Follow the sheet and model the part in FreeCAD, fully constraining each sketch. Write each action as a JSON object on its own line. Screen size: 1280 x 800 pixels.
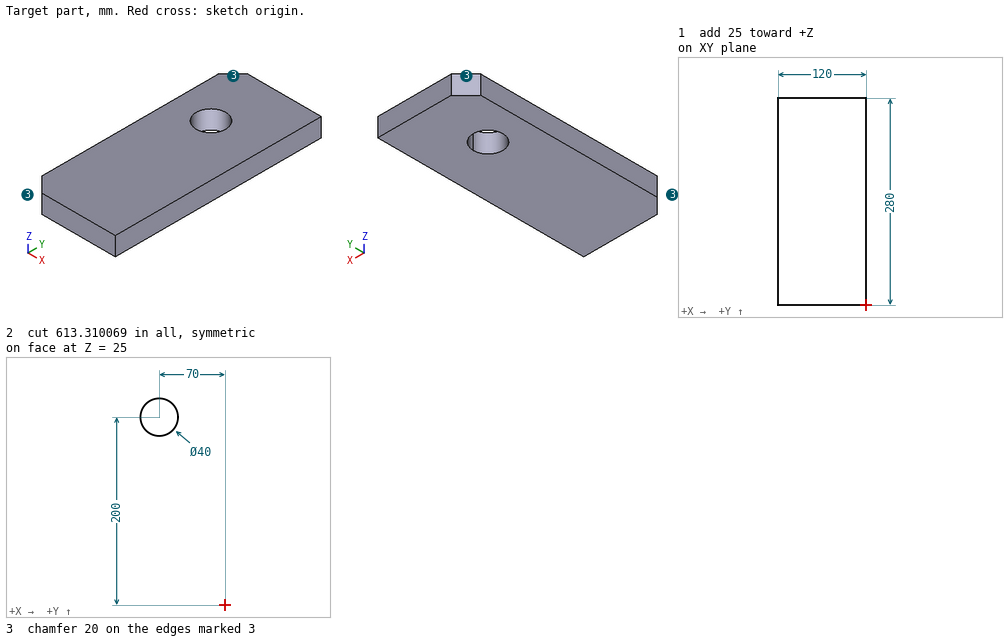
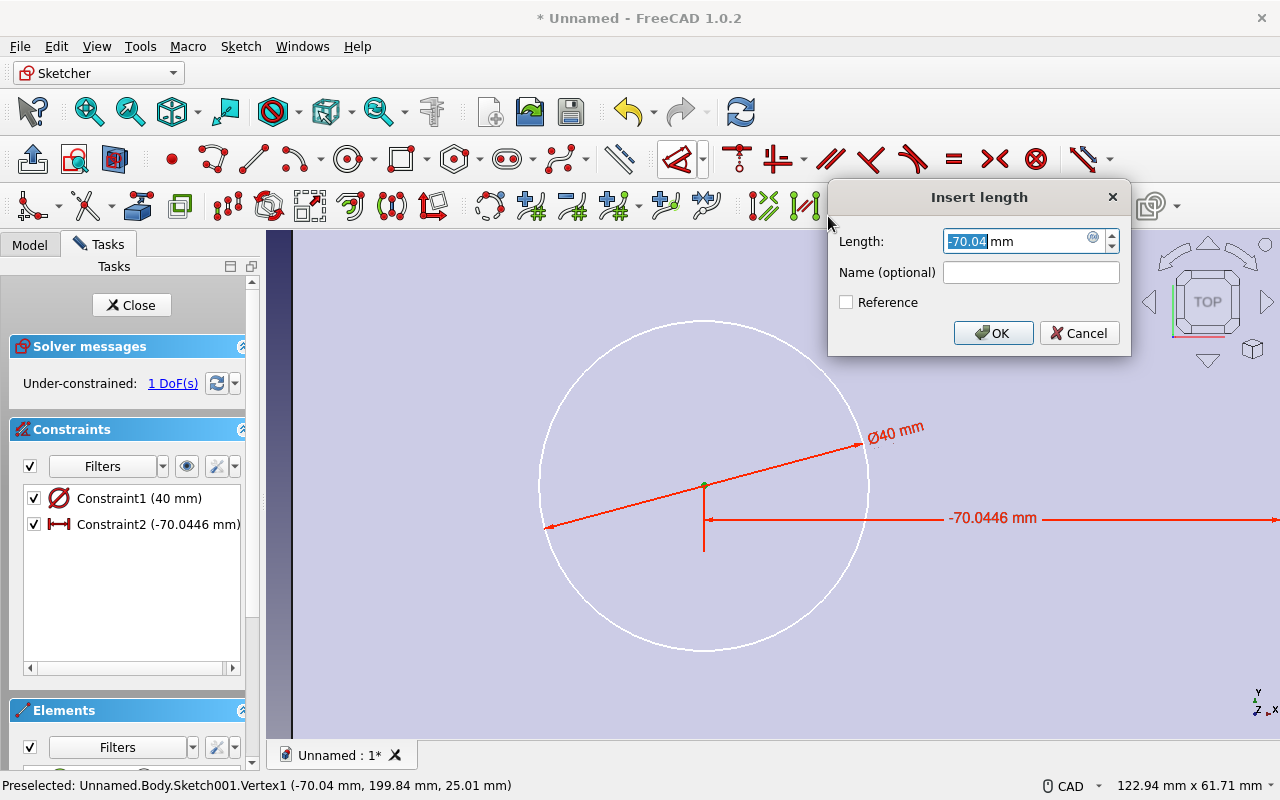
{"action": "type", "text": "-70"}
{"action": "key", "text": "Return"}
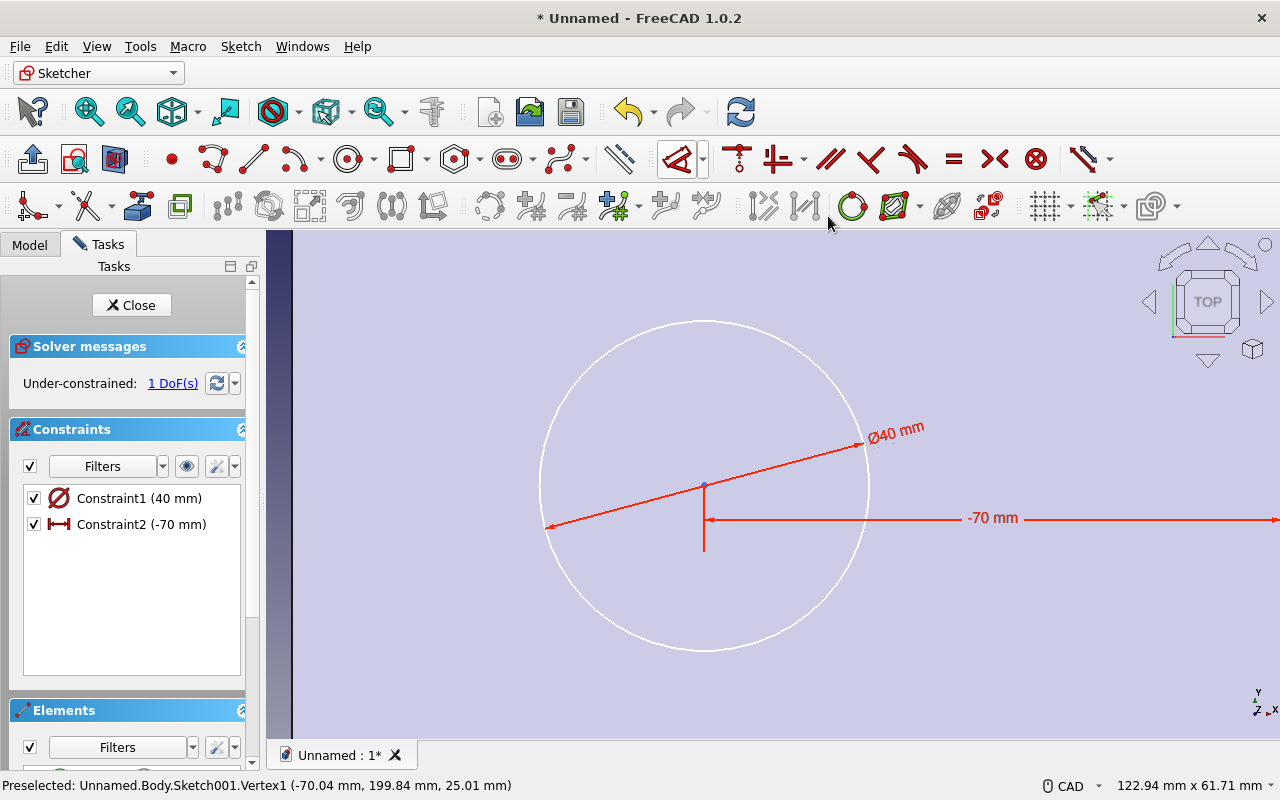
{"action": "left_click", "coordinate": [704, 486]}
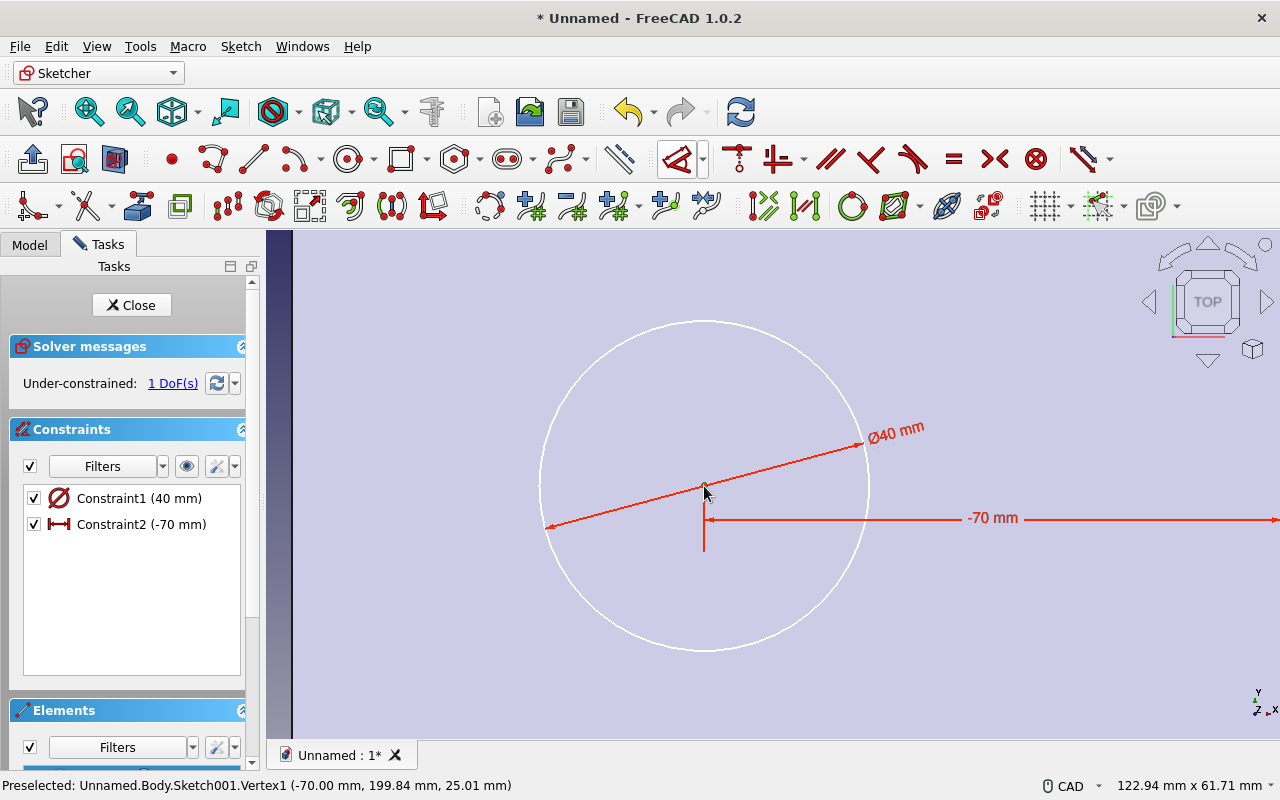
{"action": "key", "text": "i"}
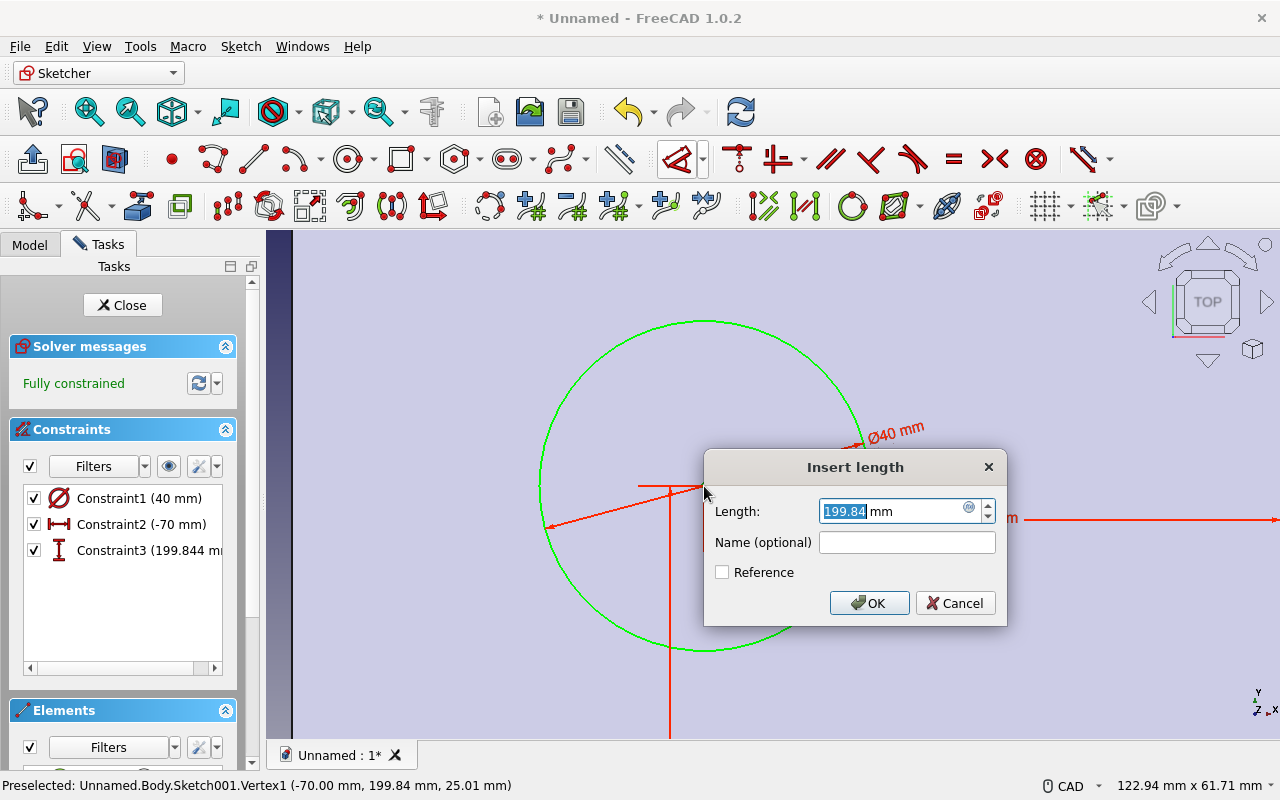
{"action": "type", "text": "200"}
{"action": "key", "text": "Return"}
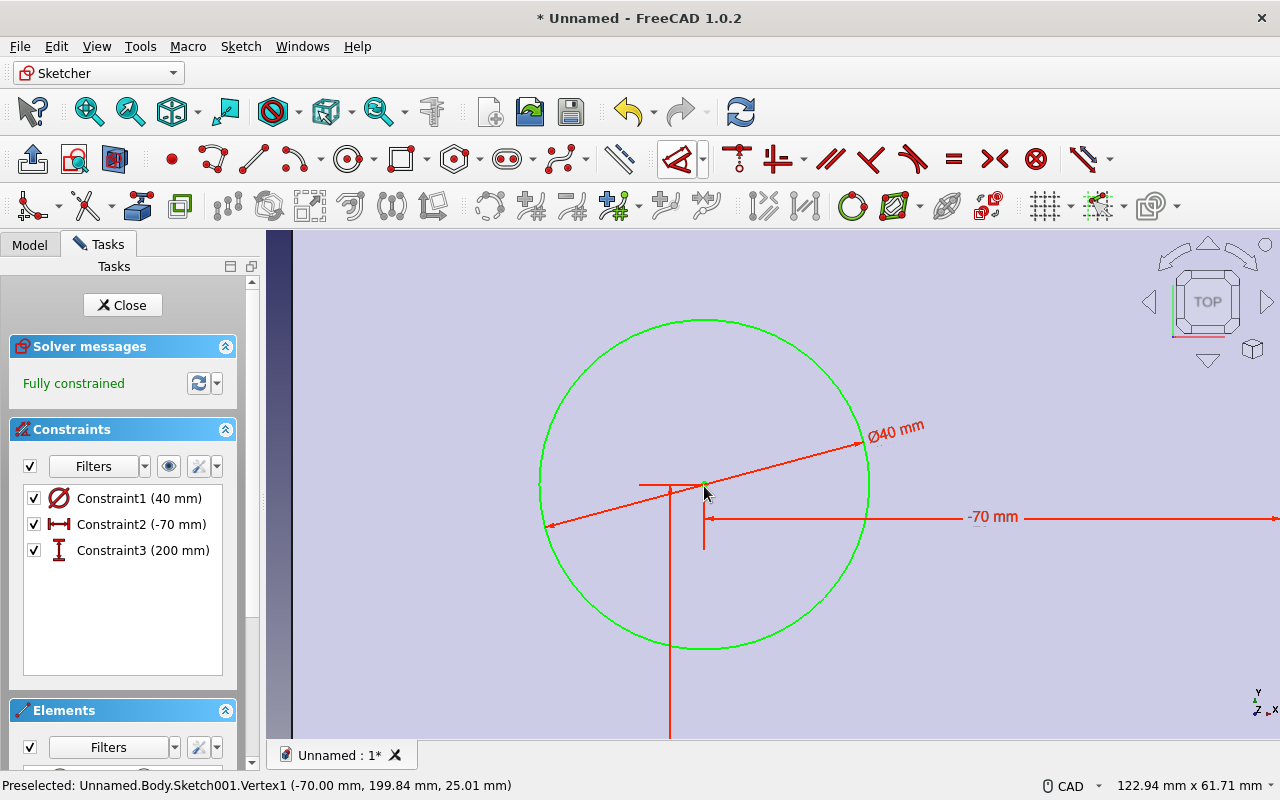
{"action": "left_click", "coordinate": [123, 305]}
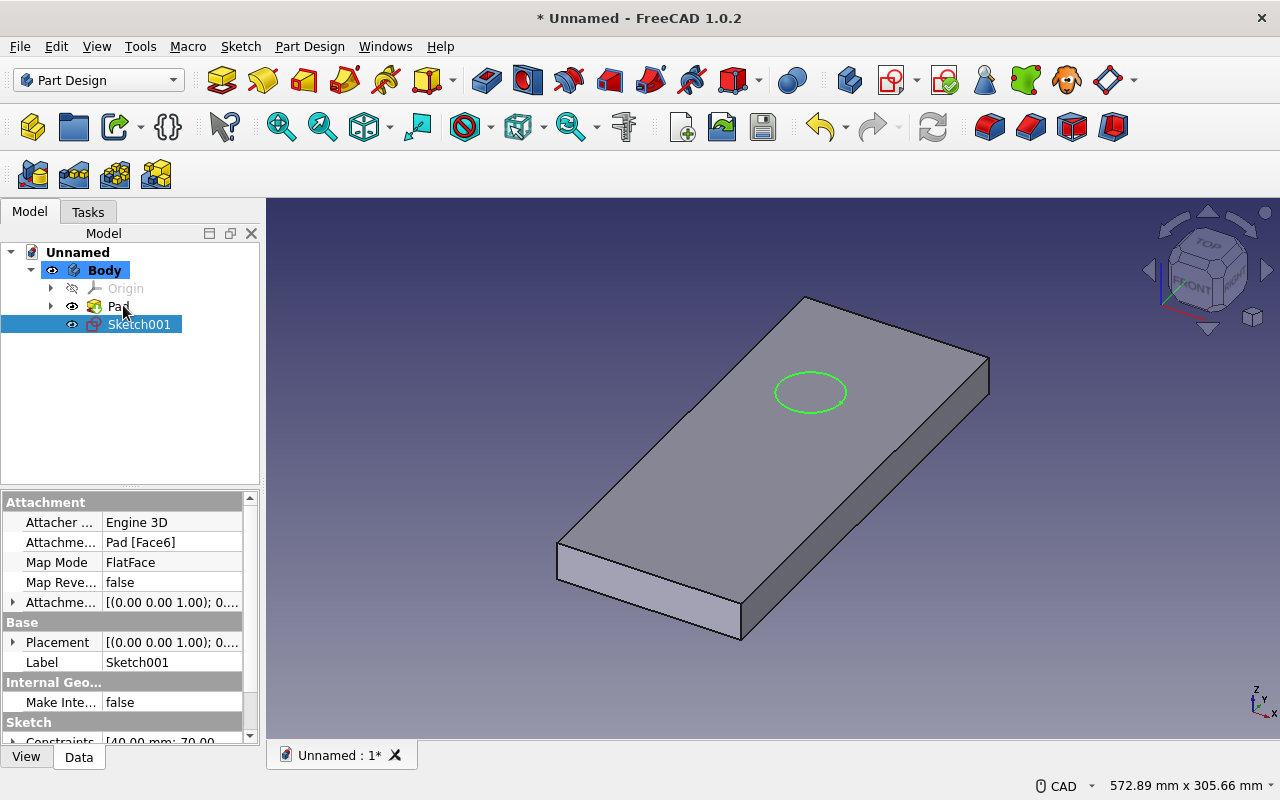
{"action": "left_click", "coordinate": [487, 80]}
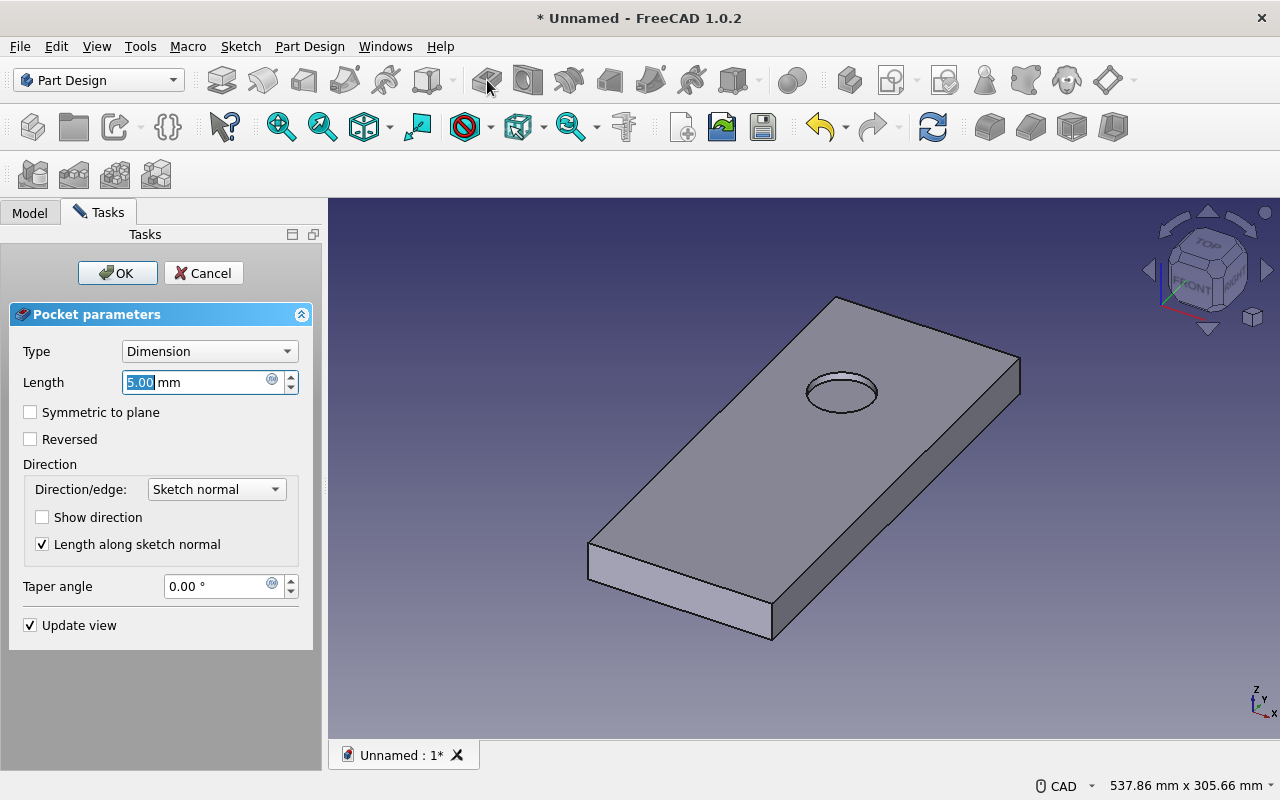
{"action": "type", "text": "613.310069"}
{"action": "key", "text": "Tab"}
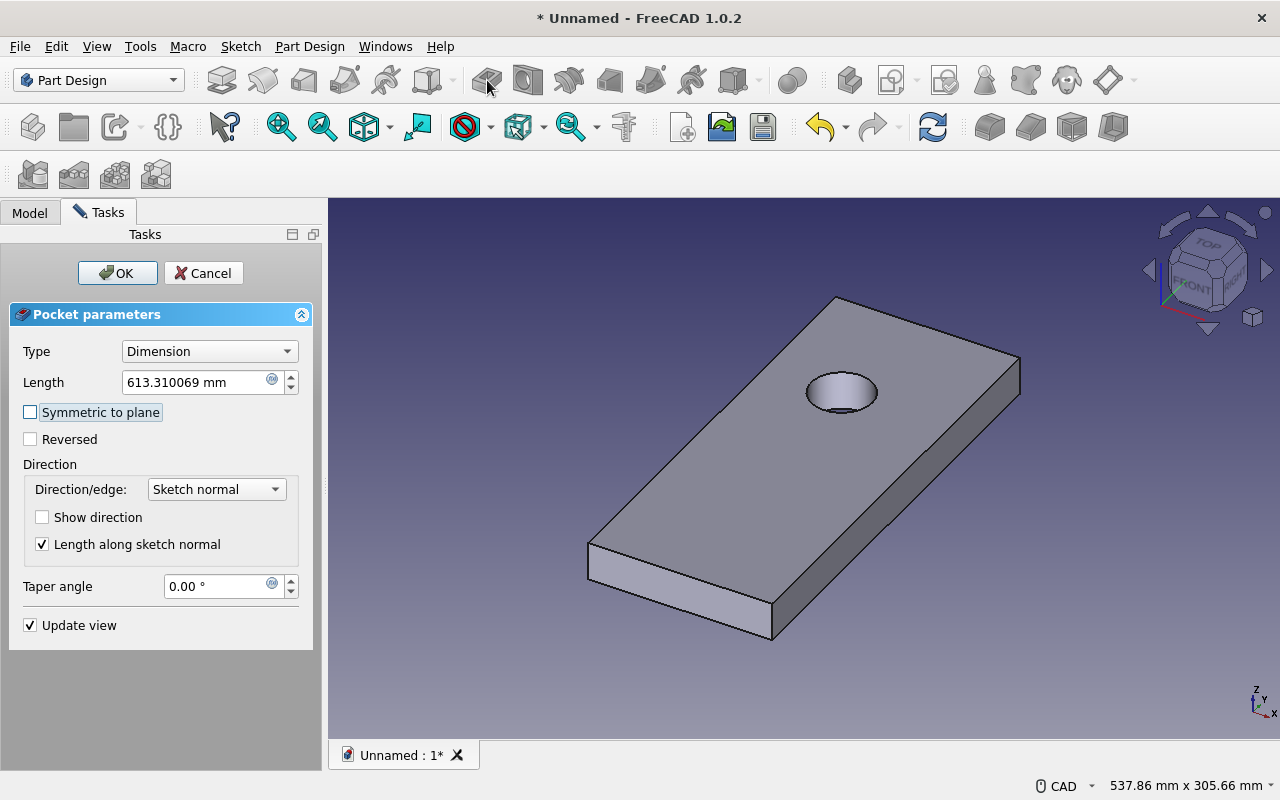
{"action": "left_click", "coordinate": [31, 412]}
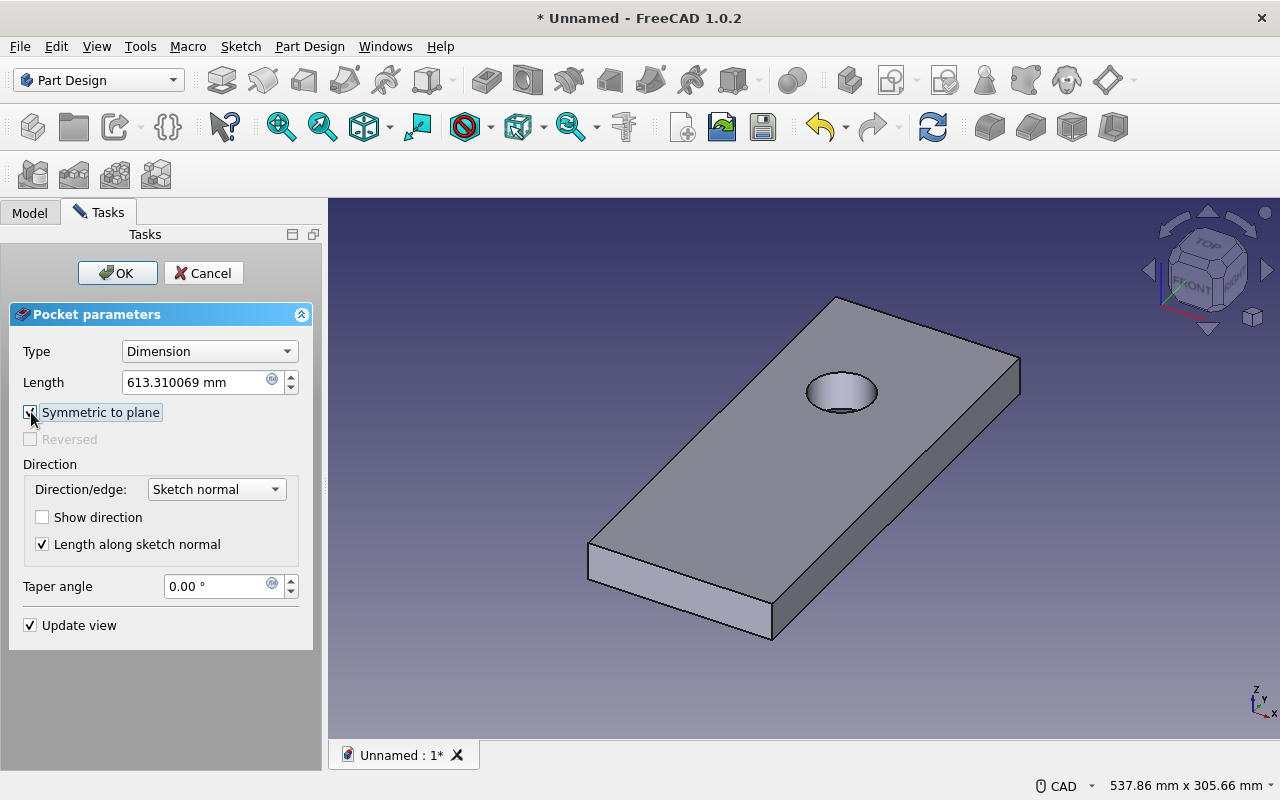
{"action": "left_click", "coordinate": [118, 273]}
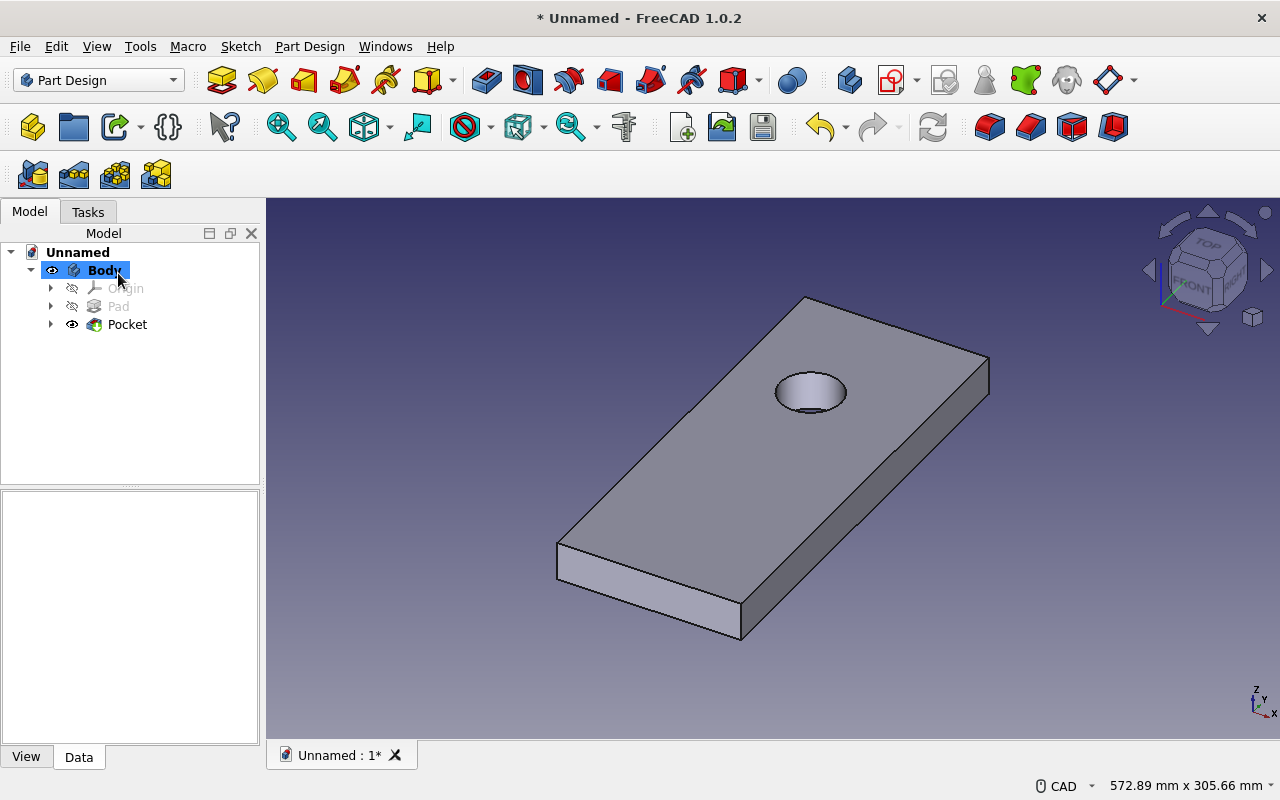
{"action": "key", "text": "0"}